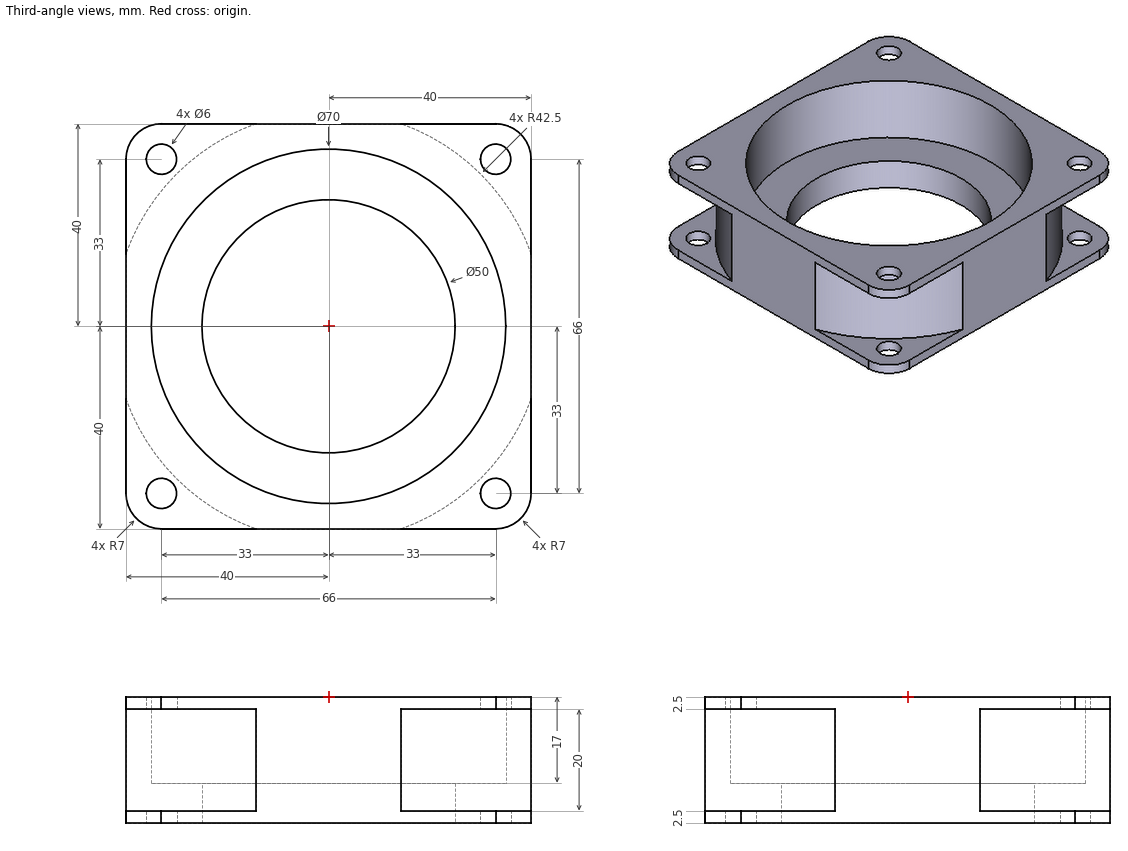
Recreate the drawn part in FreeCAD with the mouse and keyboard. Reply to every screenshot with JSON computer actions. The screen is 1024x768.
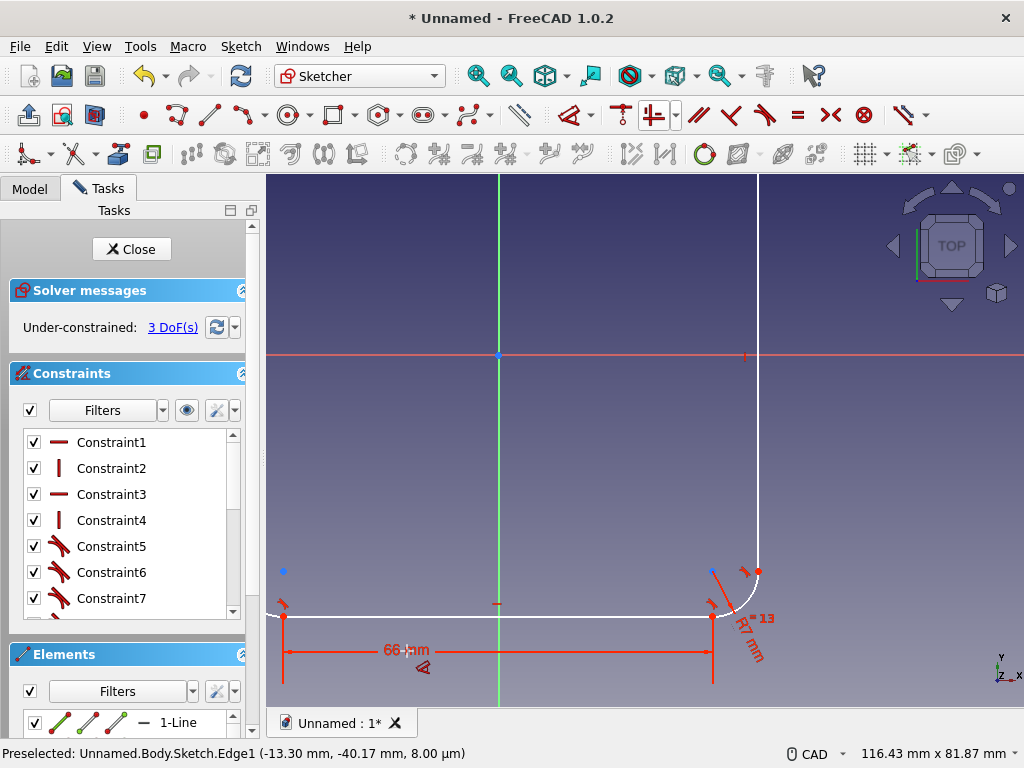
{"action": "left_click", "coordinate": [758, 442]}
{"action": "left_click", "coordinate": [792, 387]}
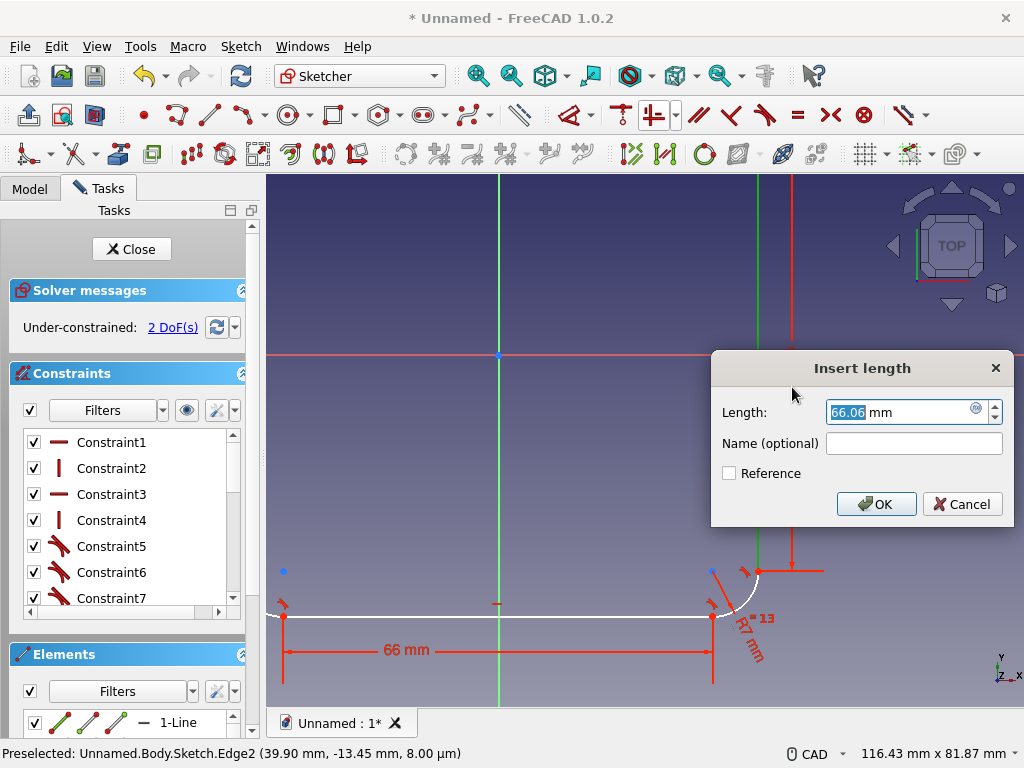
{"action": "type", "text": "66"}
{"action": "key", "text": "Return"}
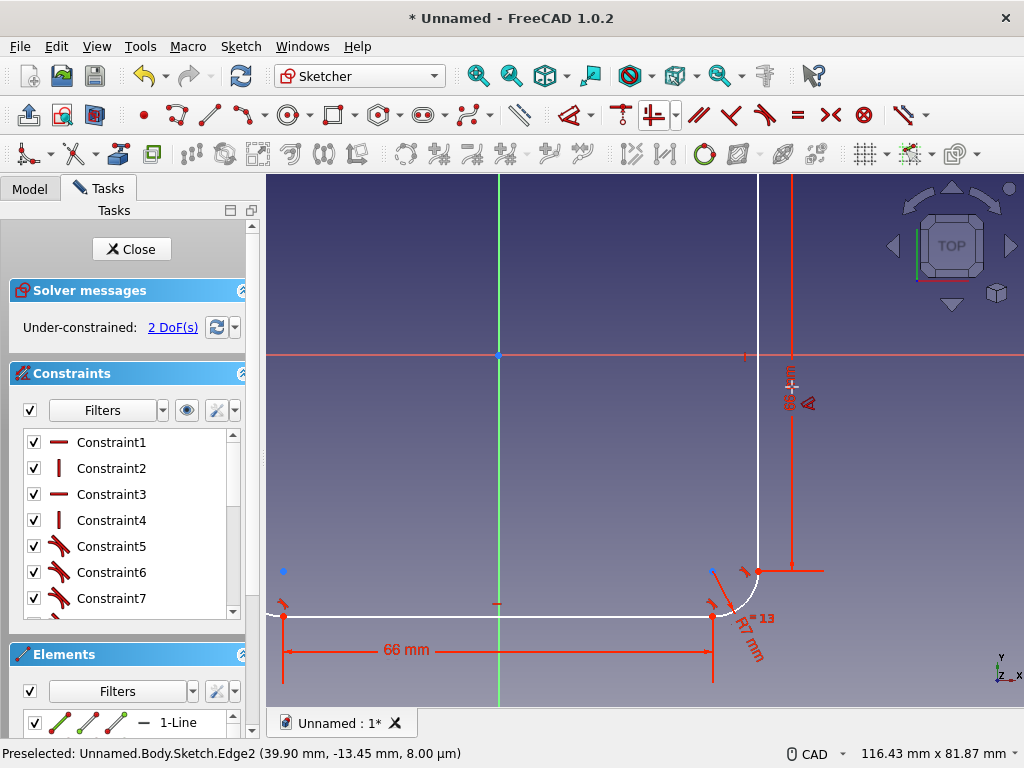
{"action": "scroll", "coordinate": [735, 613], "scroll_direction": "down", "scroll_amount": 2}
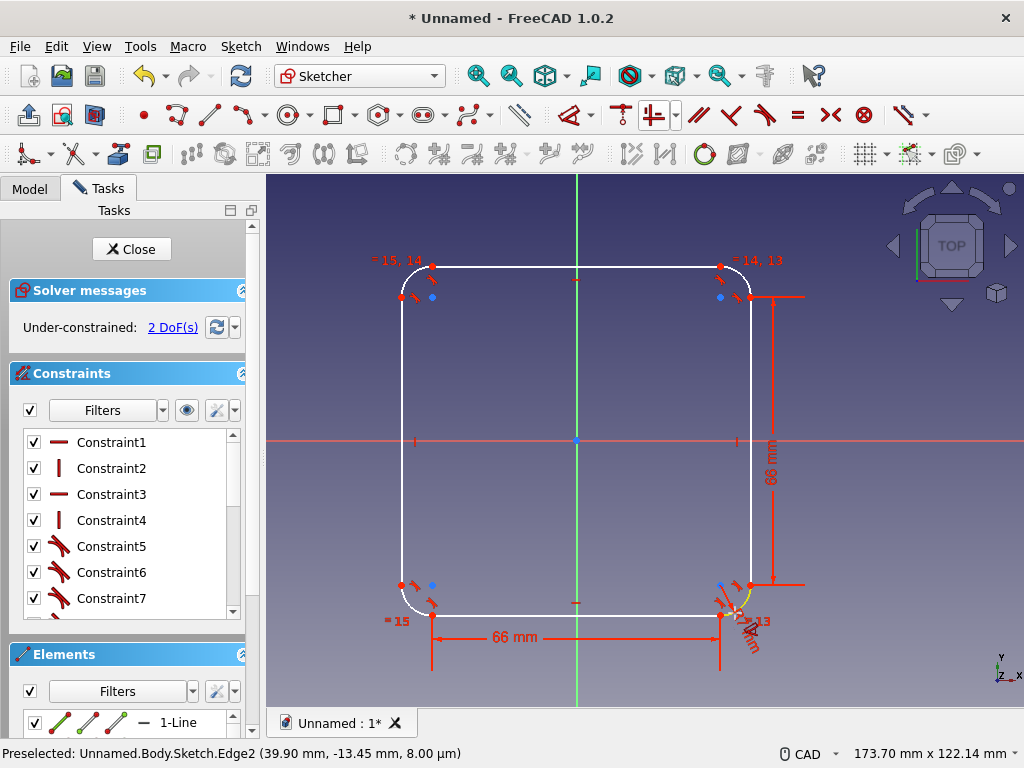
{"action": "left_click", "coordinate": [432, 616]}
{"action": "left_click", "coordinate": [505, 407]}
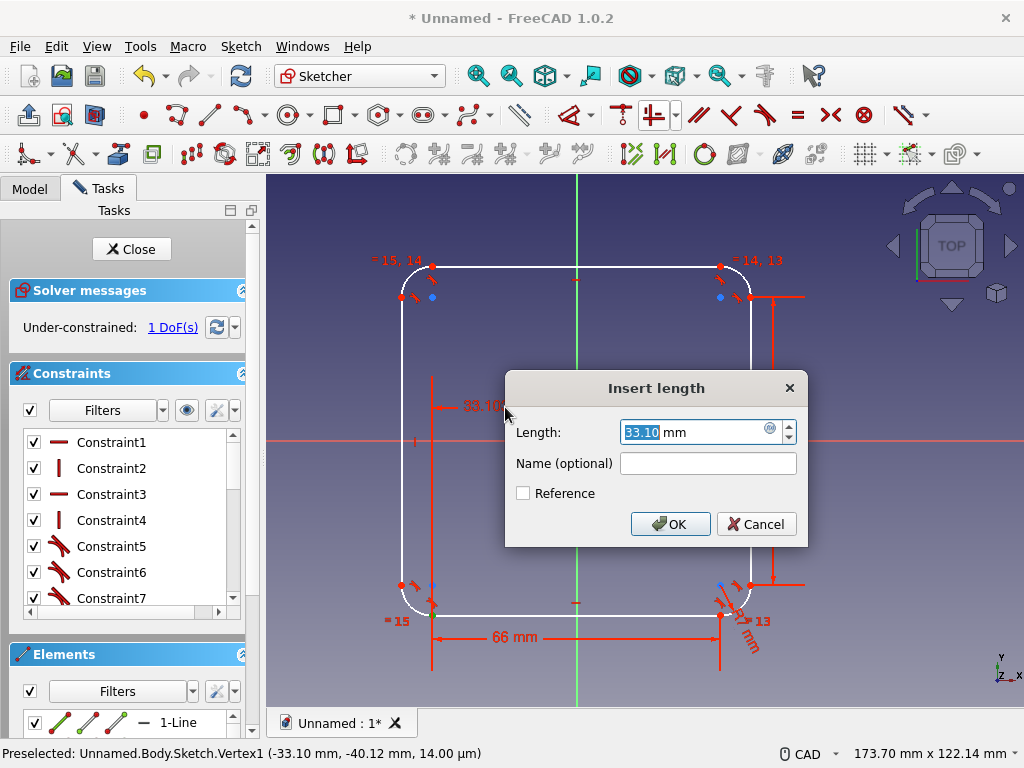
{"action": "type", "text": "33"}
{"action": "key", "text": "Return"}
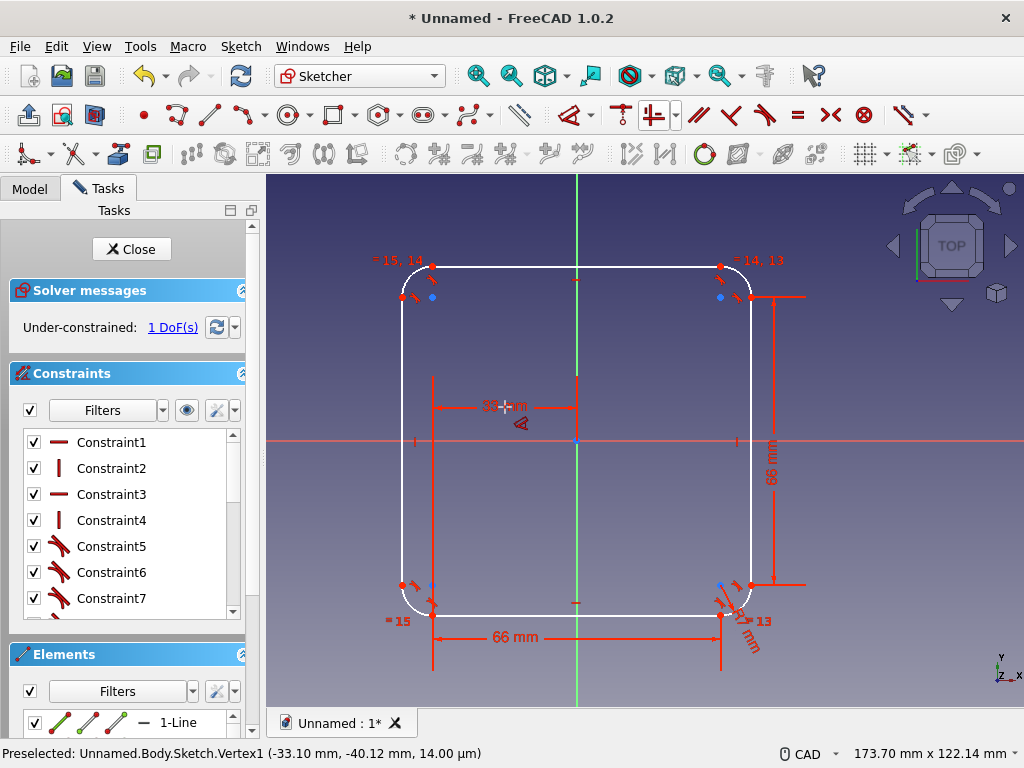
{"action": "left_click", "coordinate": [433, 616]}
{"action": "left_click", "coordinate": [611, 528]}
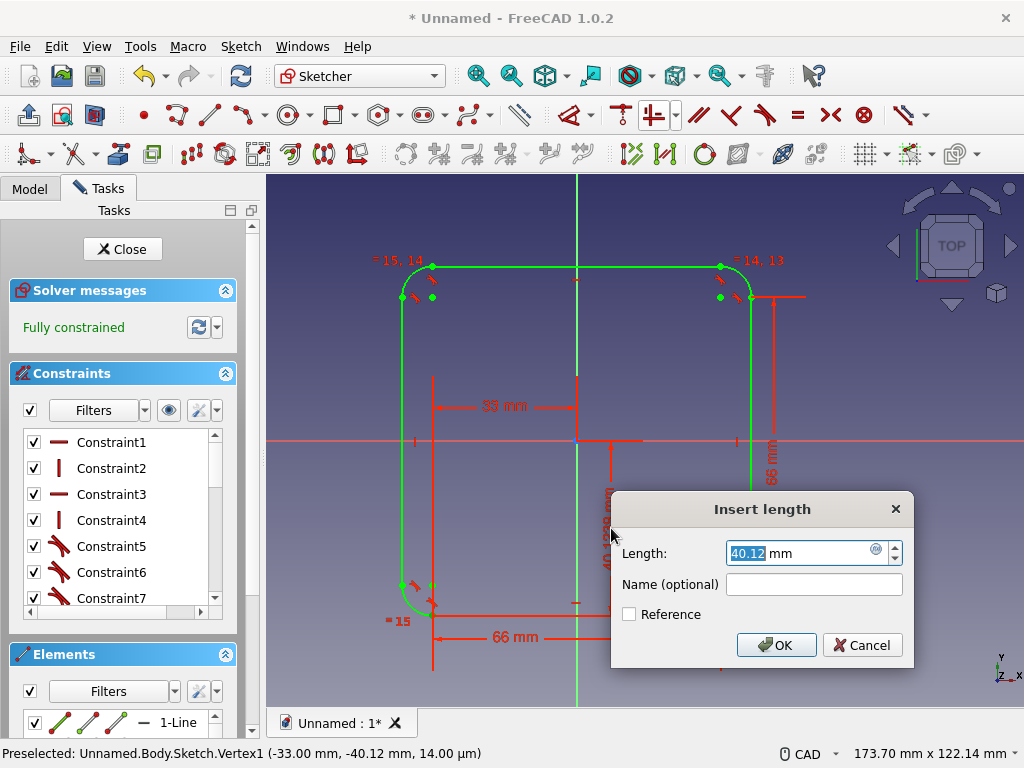
{"action": "type", "text": "40"}
{"action": "key", "text": "Return"}
{"action": "key", "text": "Escape"}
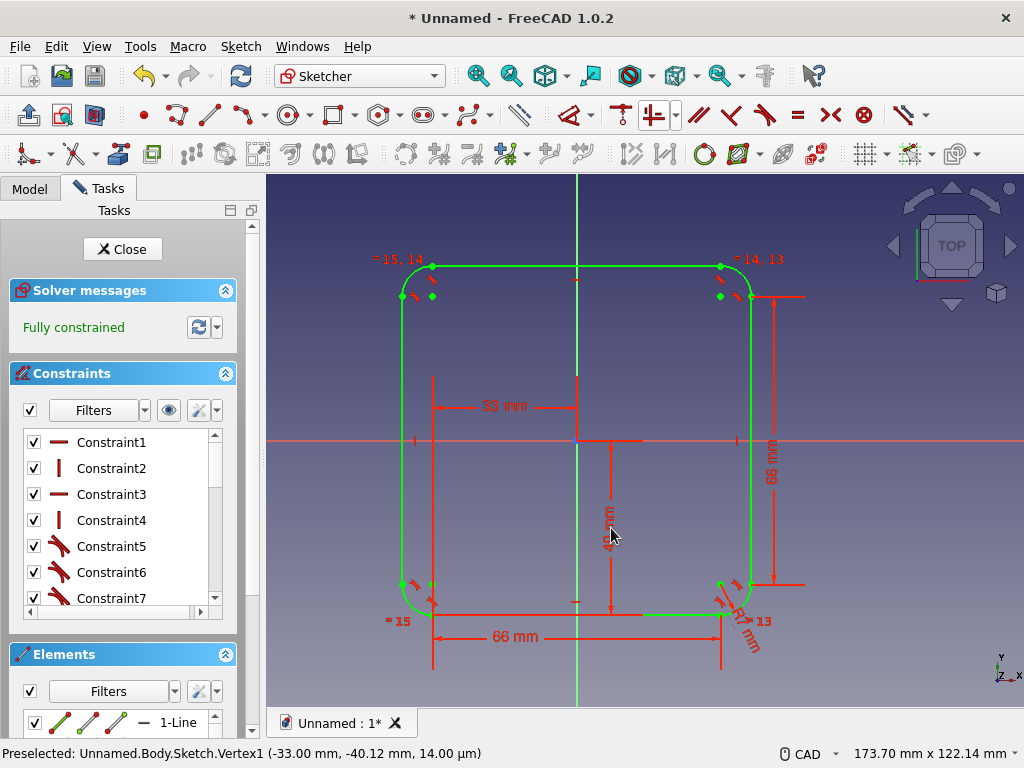
{"action": "left_click", "coordinate": [123, 249]}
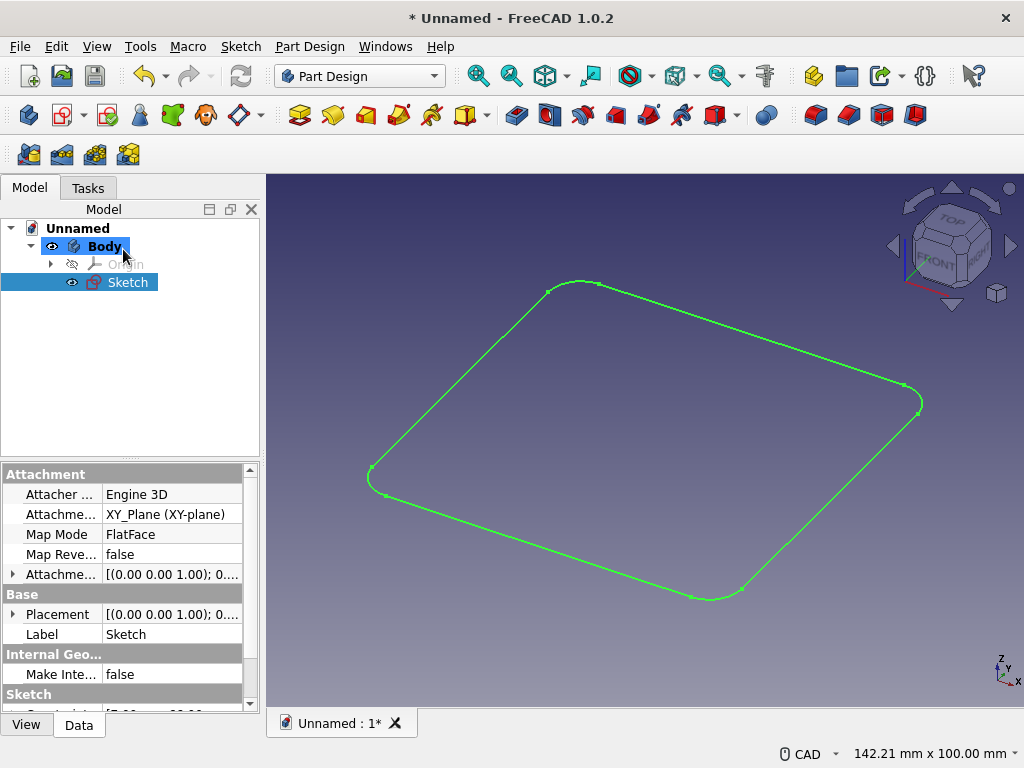
{"action": "left_click", "coordinate": [300, 116]}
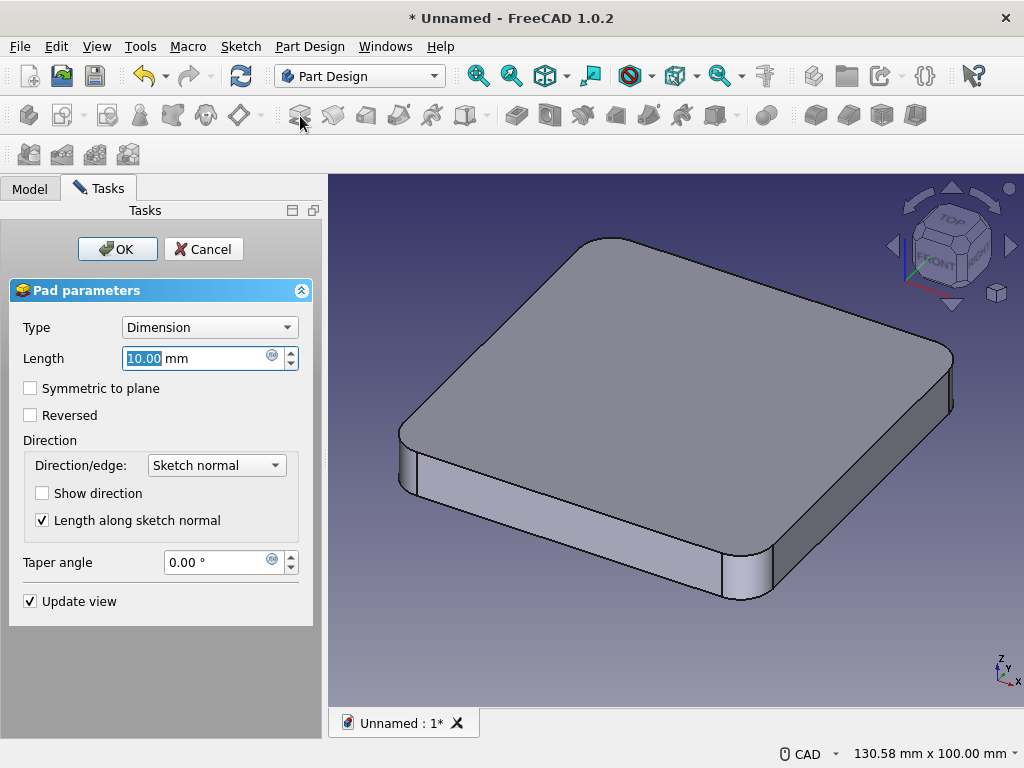
{"action": "type", "text": "2.5"}
{"action": "key", "text": "Tab"}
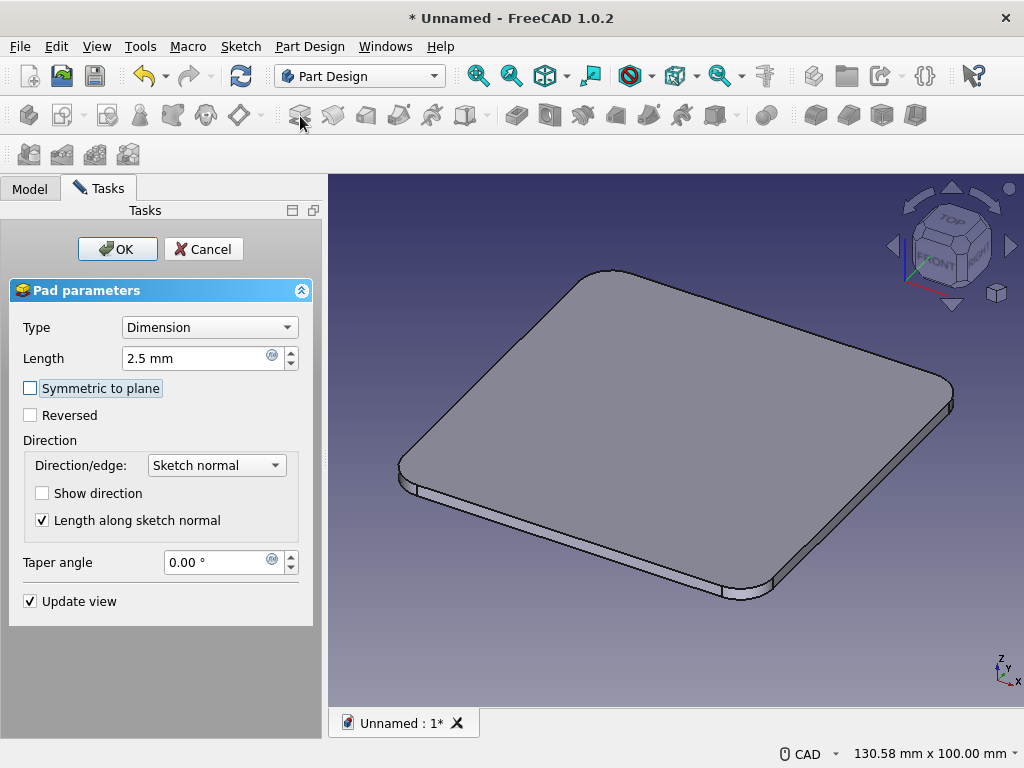
{"action": "left_click", "coordinate": [31, 415]}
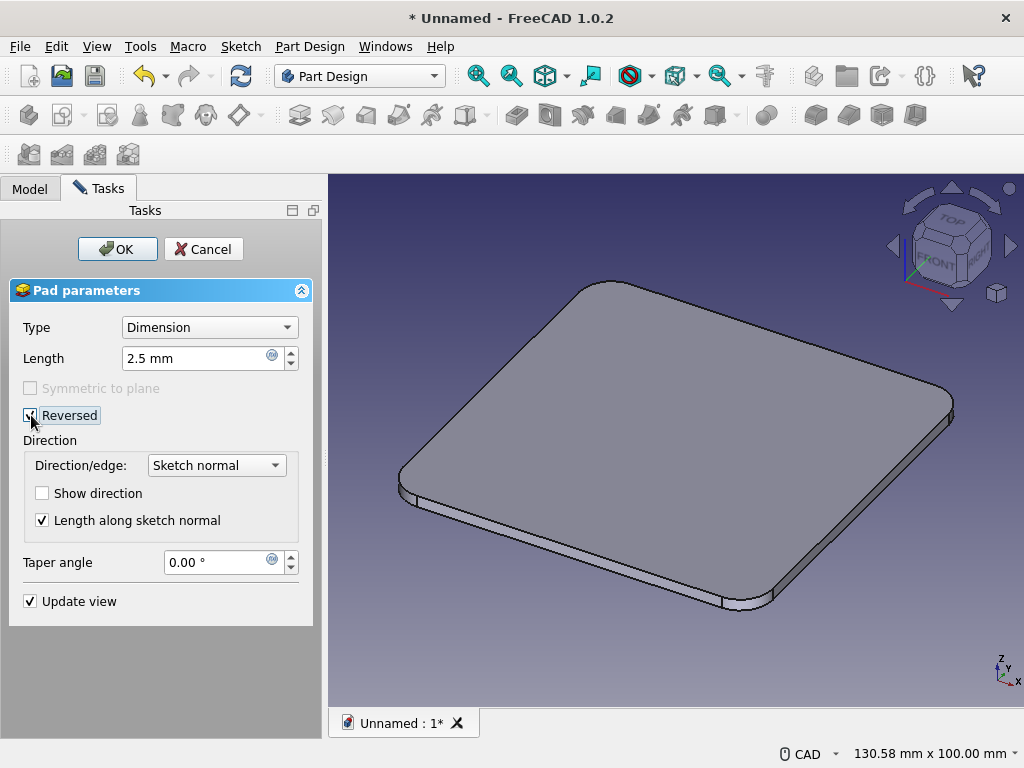
{"action": "left_click", "coordinate": [118, 249]}